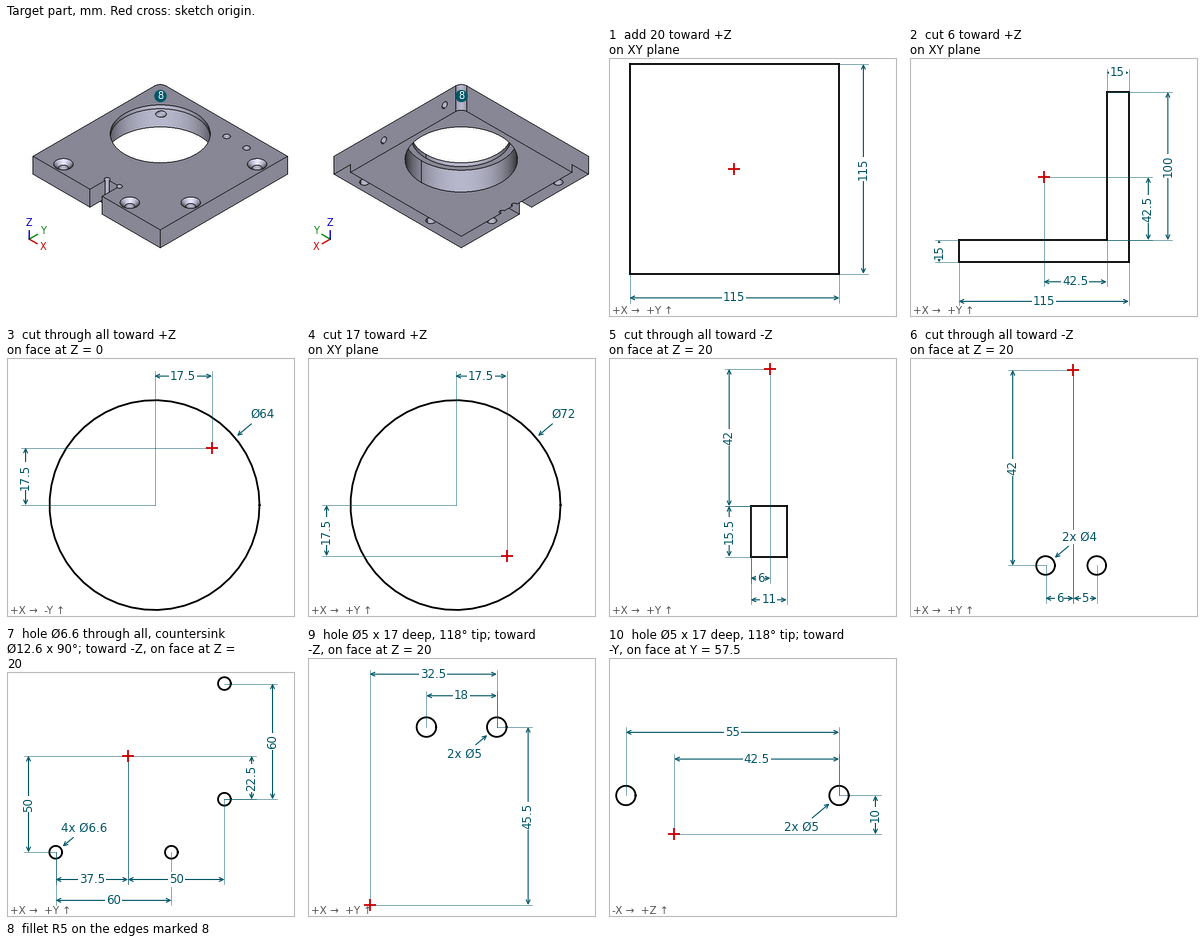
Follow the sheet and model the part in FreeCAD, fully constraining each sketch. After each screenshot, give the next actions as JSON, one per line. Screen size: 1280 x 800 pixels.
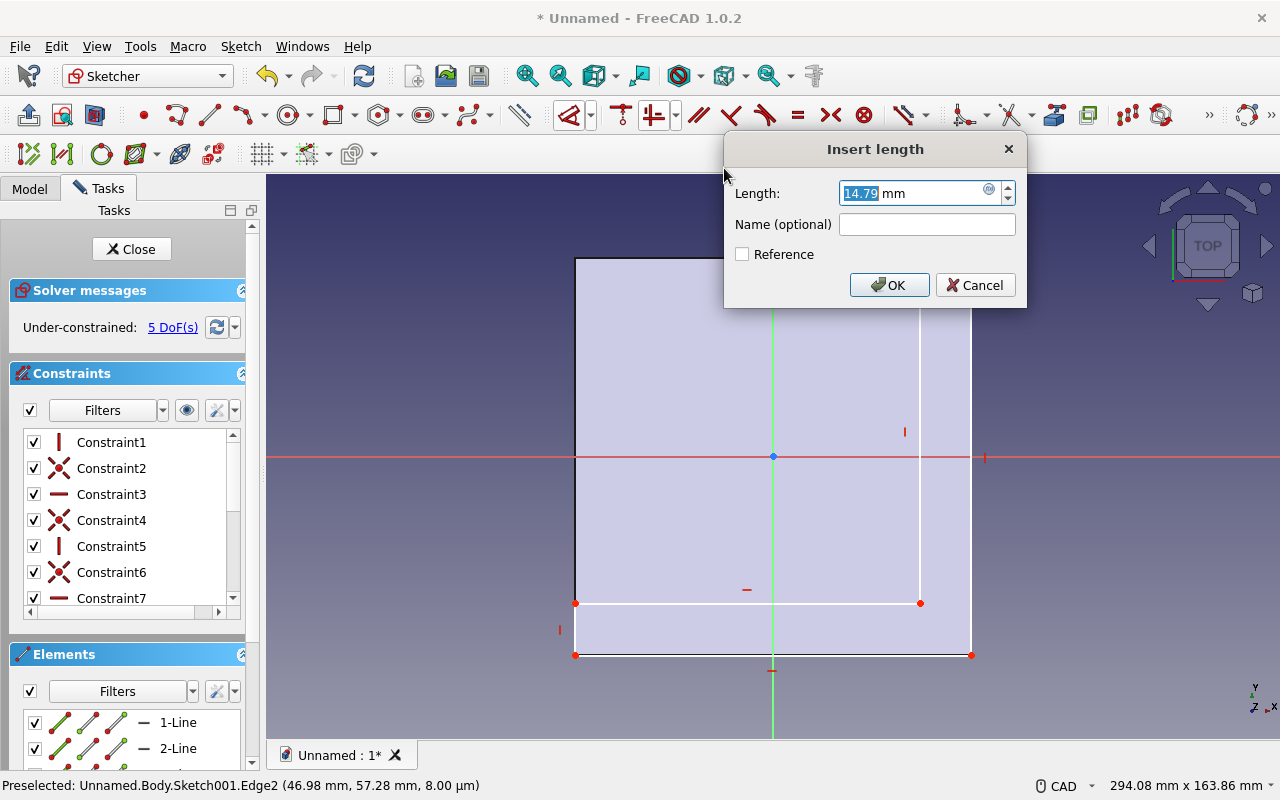
{"action": "type", "text": "15"}
{"action": "key", "text": "Return"}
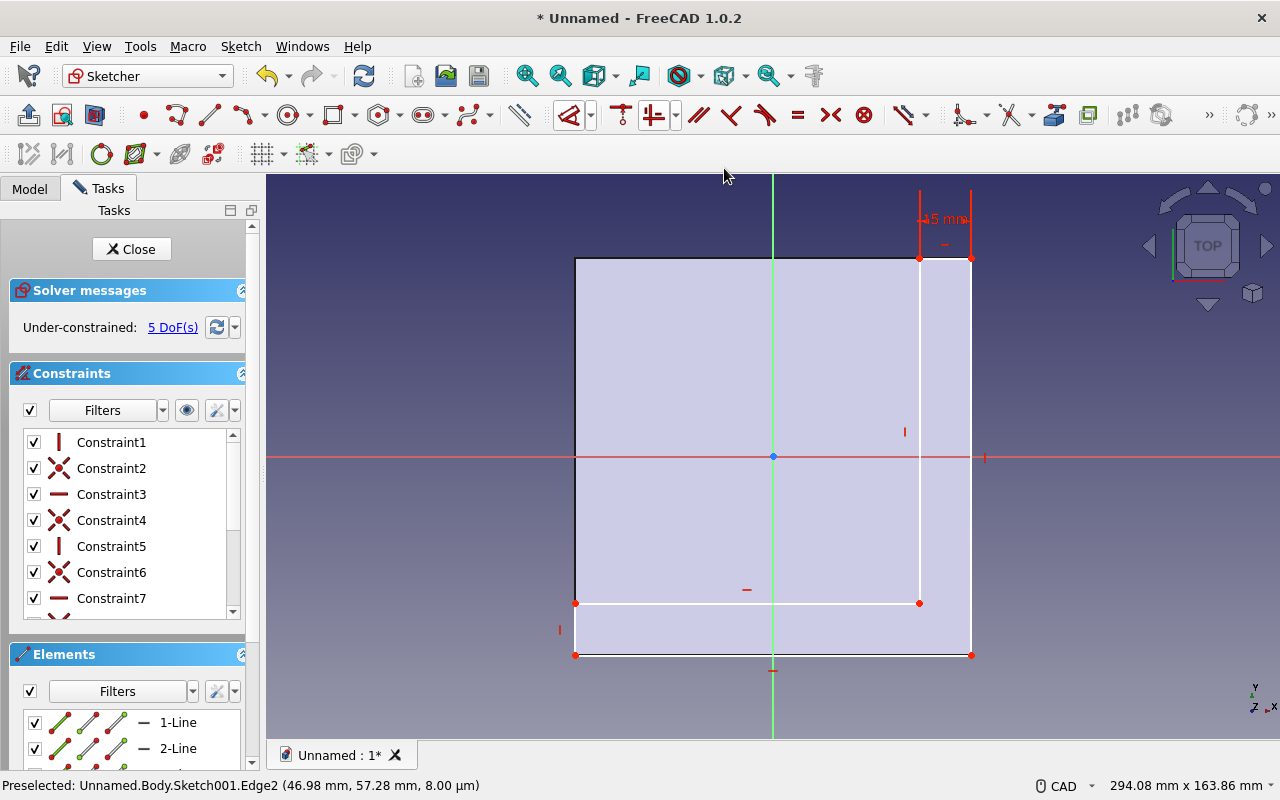
{"action": "left_click", "coordinate": [575, 640]}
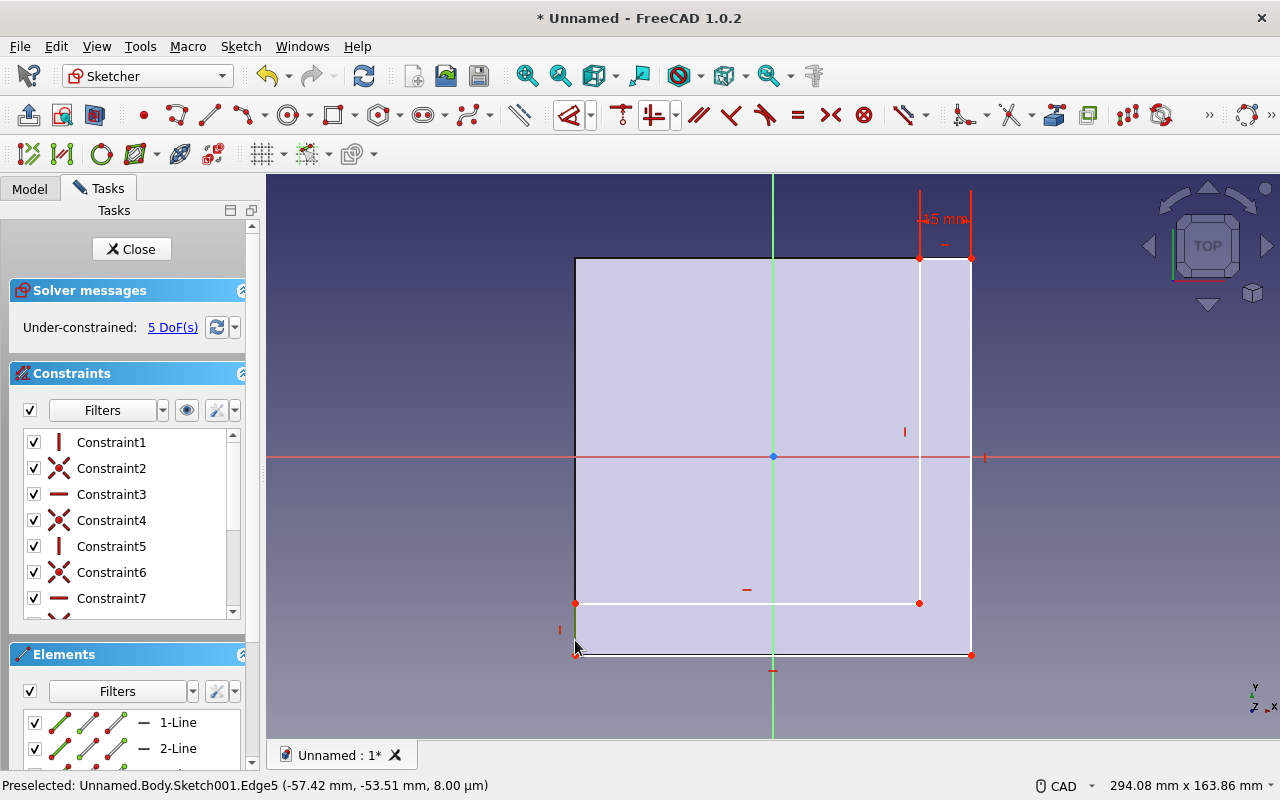
{"action": "key", "text": "i"}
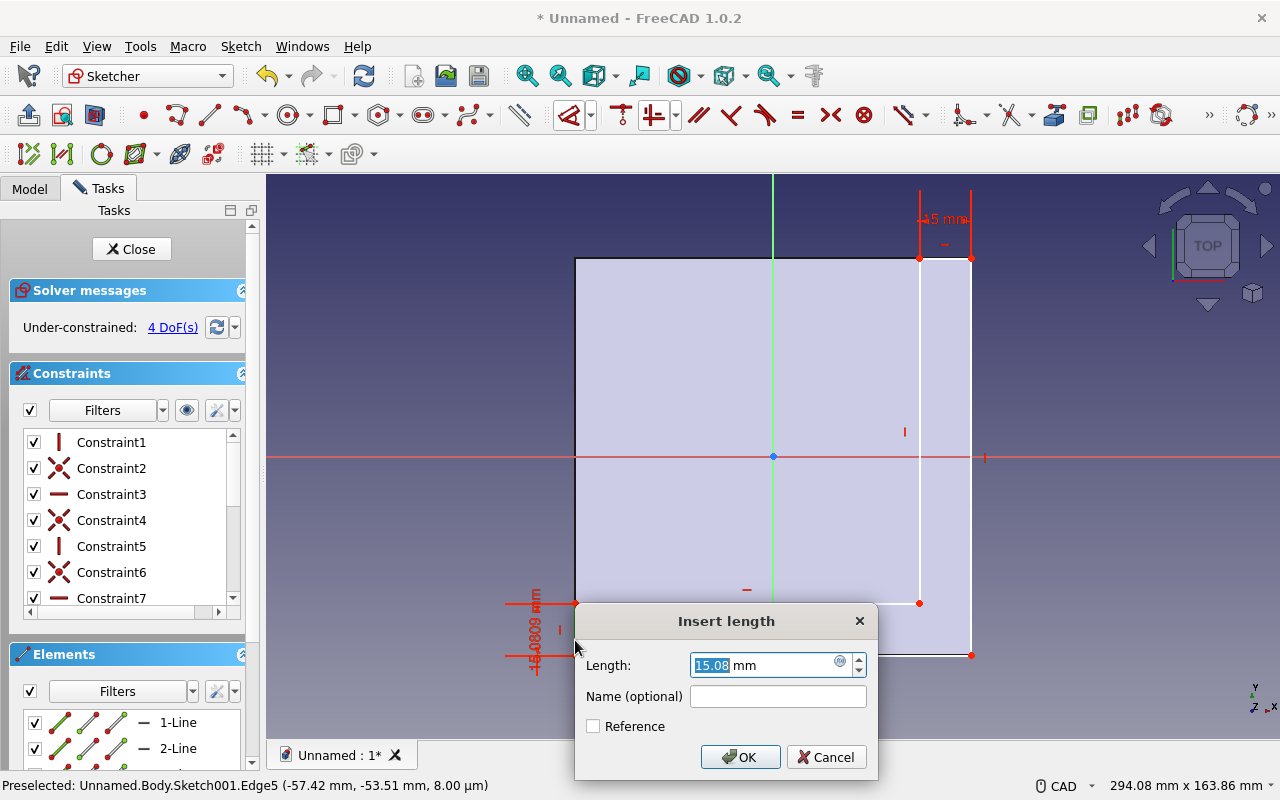
{"action": "type", "text": "15"}
{"action": "key", "text": "Return"}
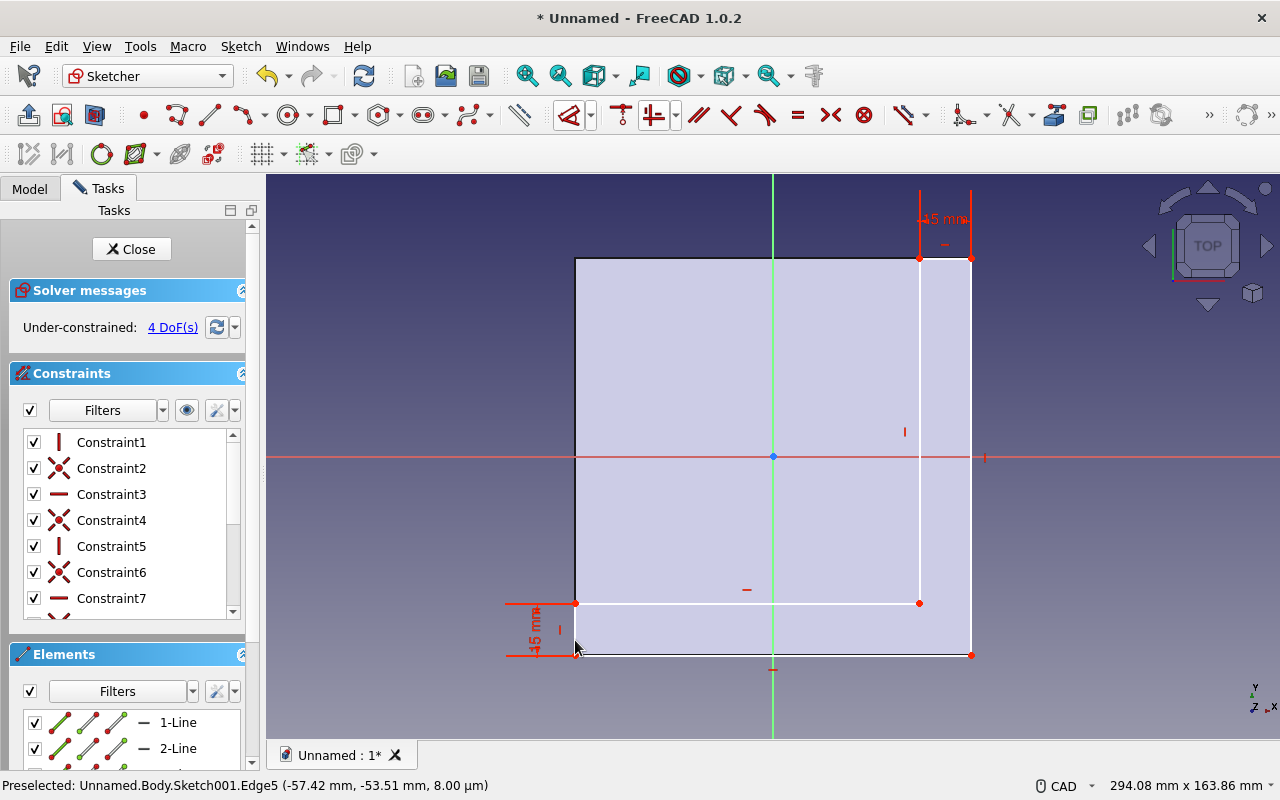
{"action": "left_click", "coordinate": [920, 500]}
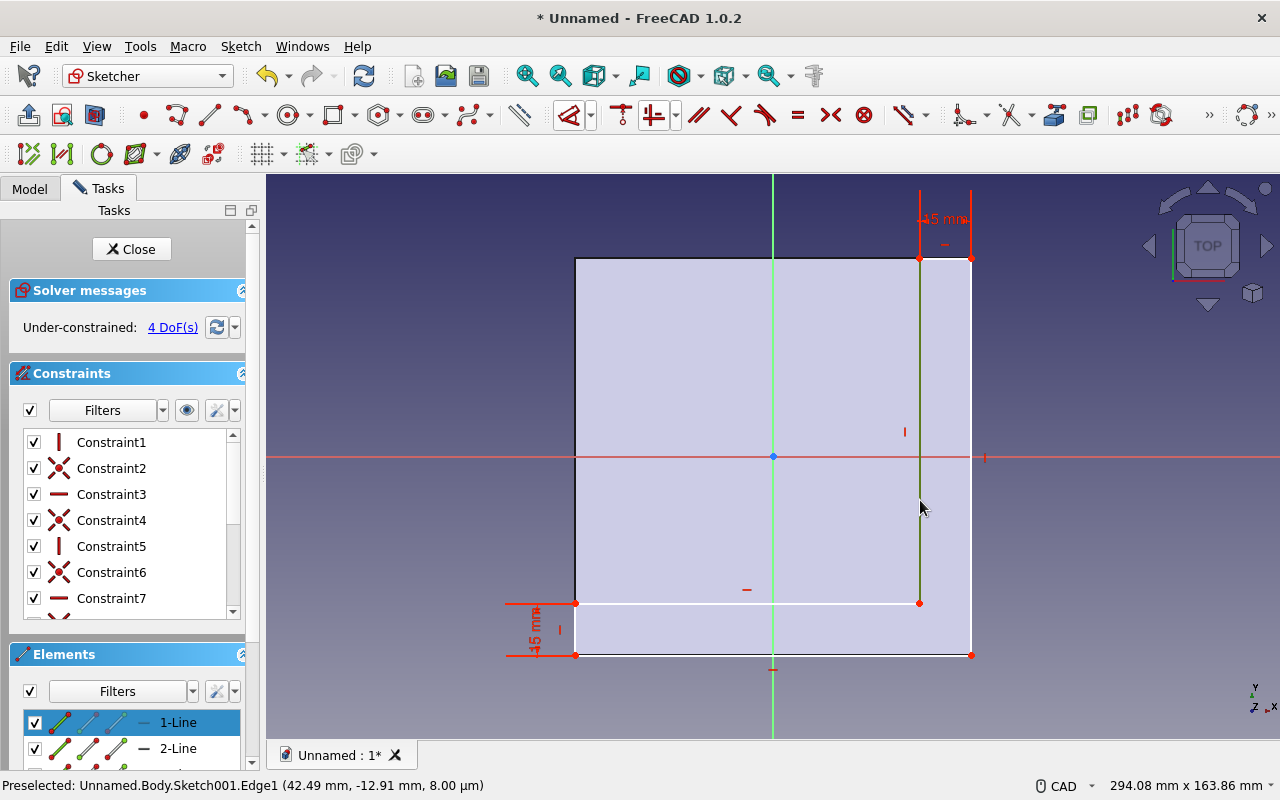
{"action": "key", "text": "i"}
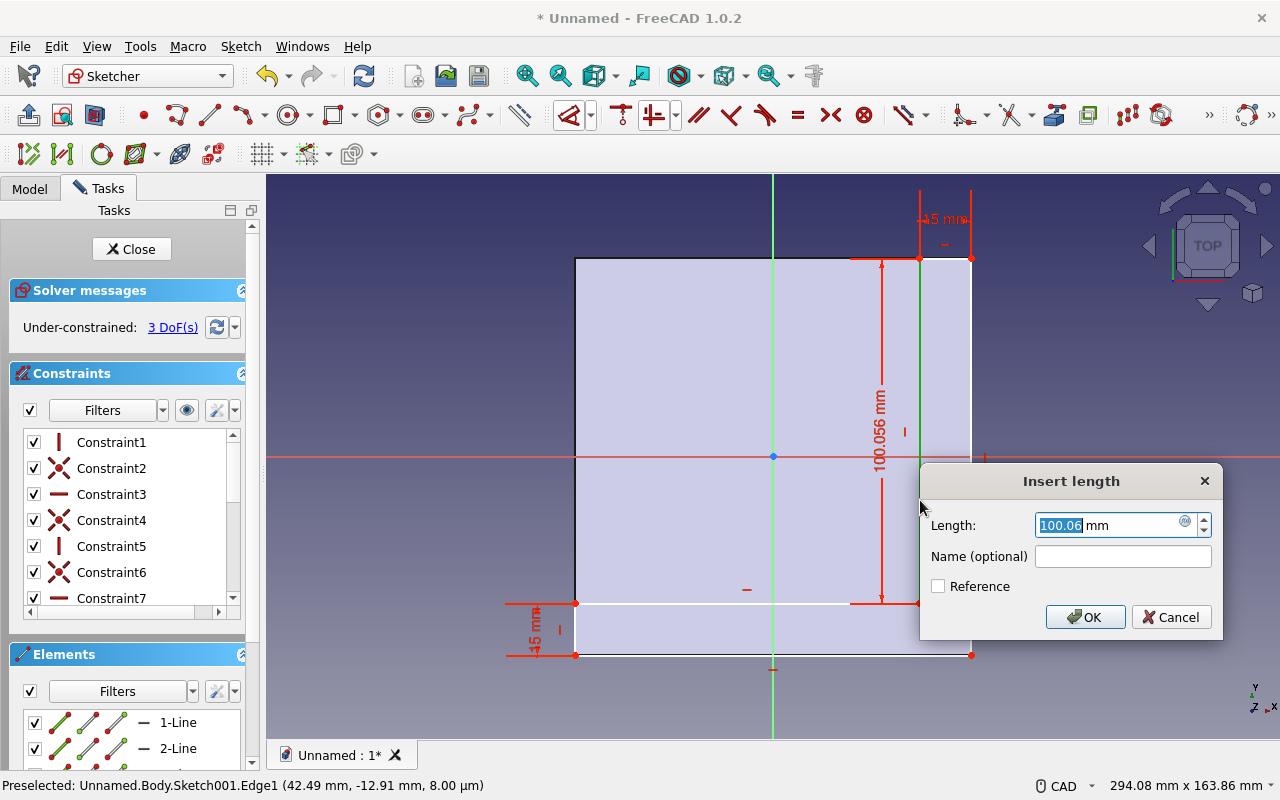
{"action": "type", "text": "100"}
{"action": "key", "text": "Return"}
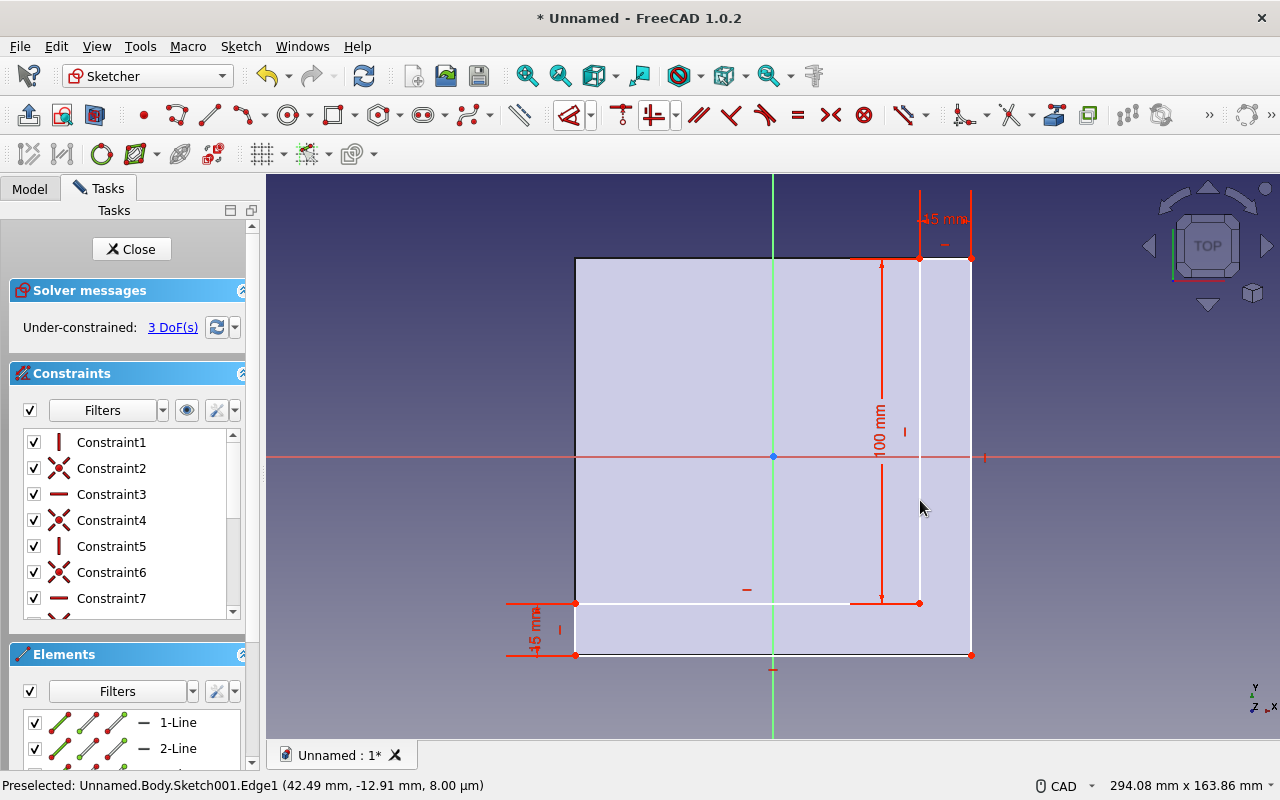
{"action": "left_click", "coordinate": [852, 656]}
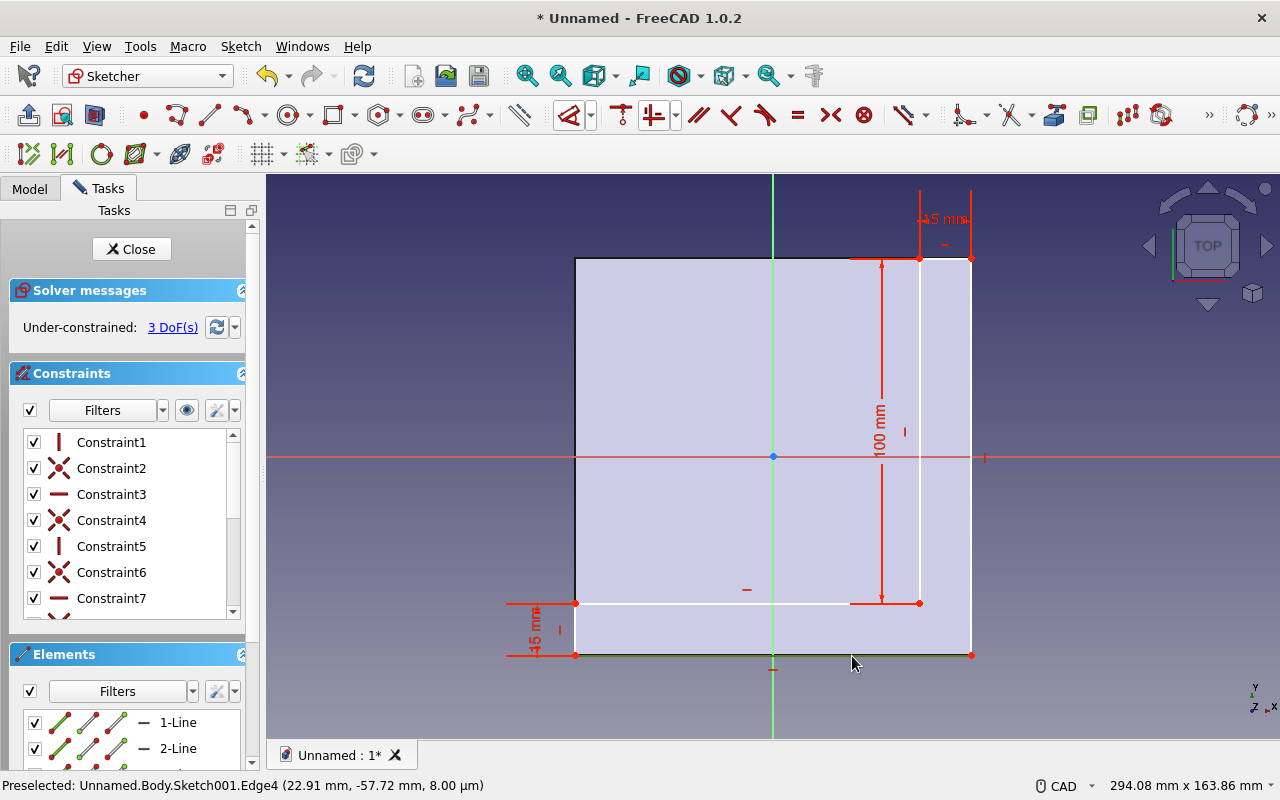
{"action": "key", "text": "l"}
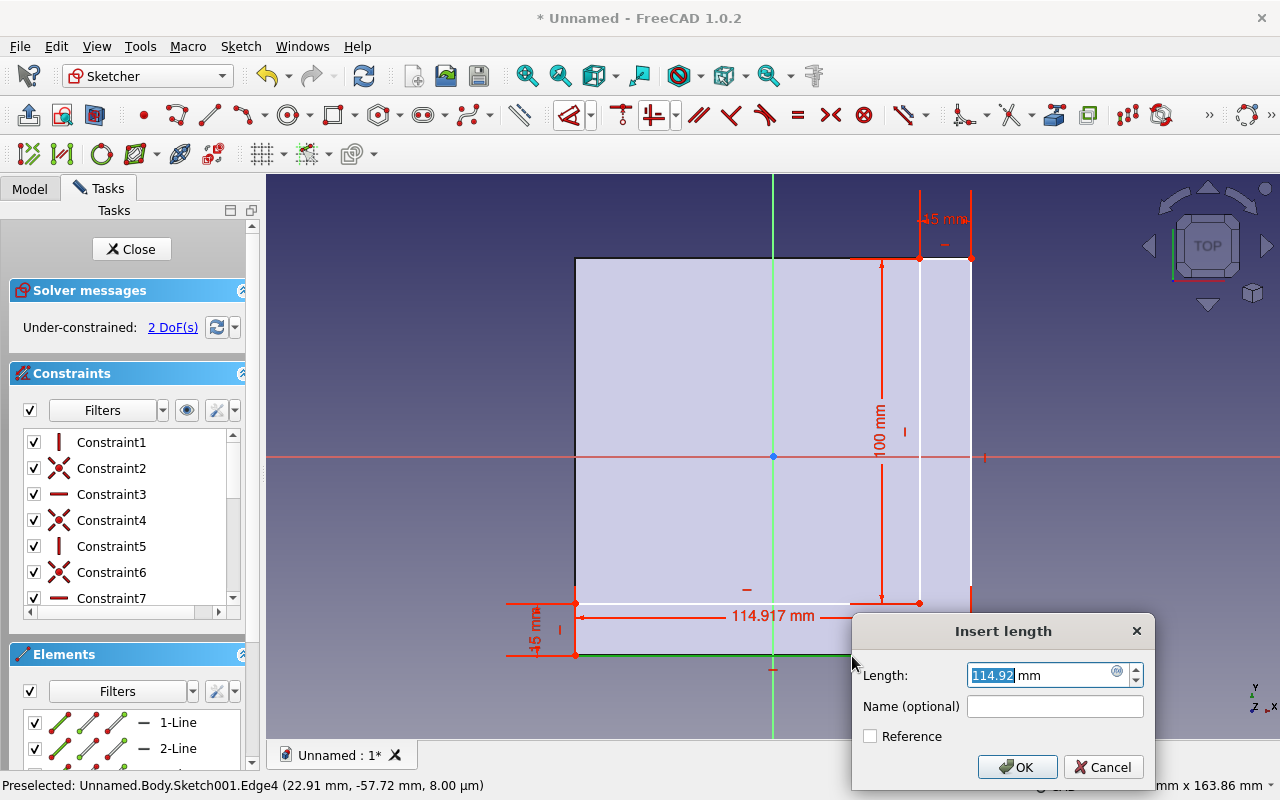
{"action": "type", "text": "115"}
{"action": "key", "text": "Return"}